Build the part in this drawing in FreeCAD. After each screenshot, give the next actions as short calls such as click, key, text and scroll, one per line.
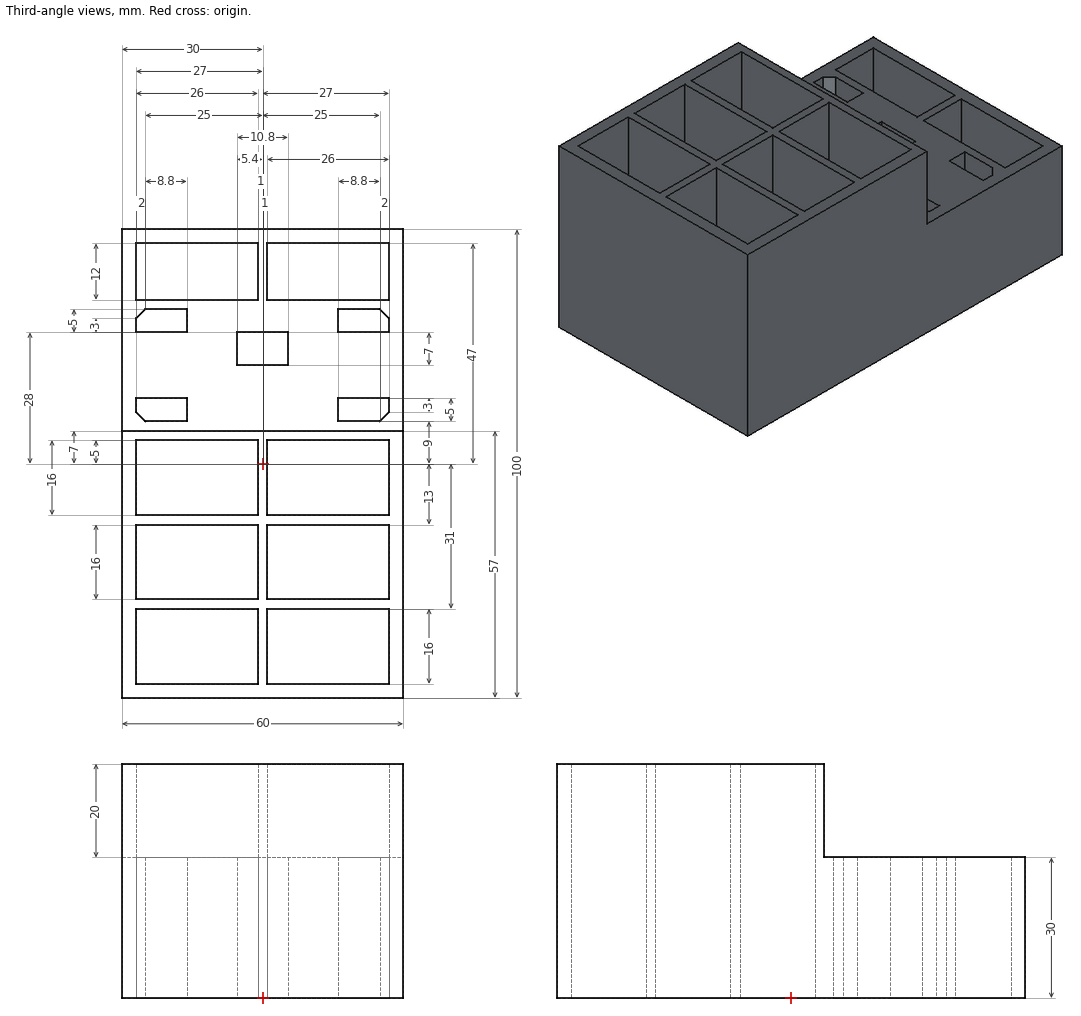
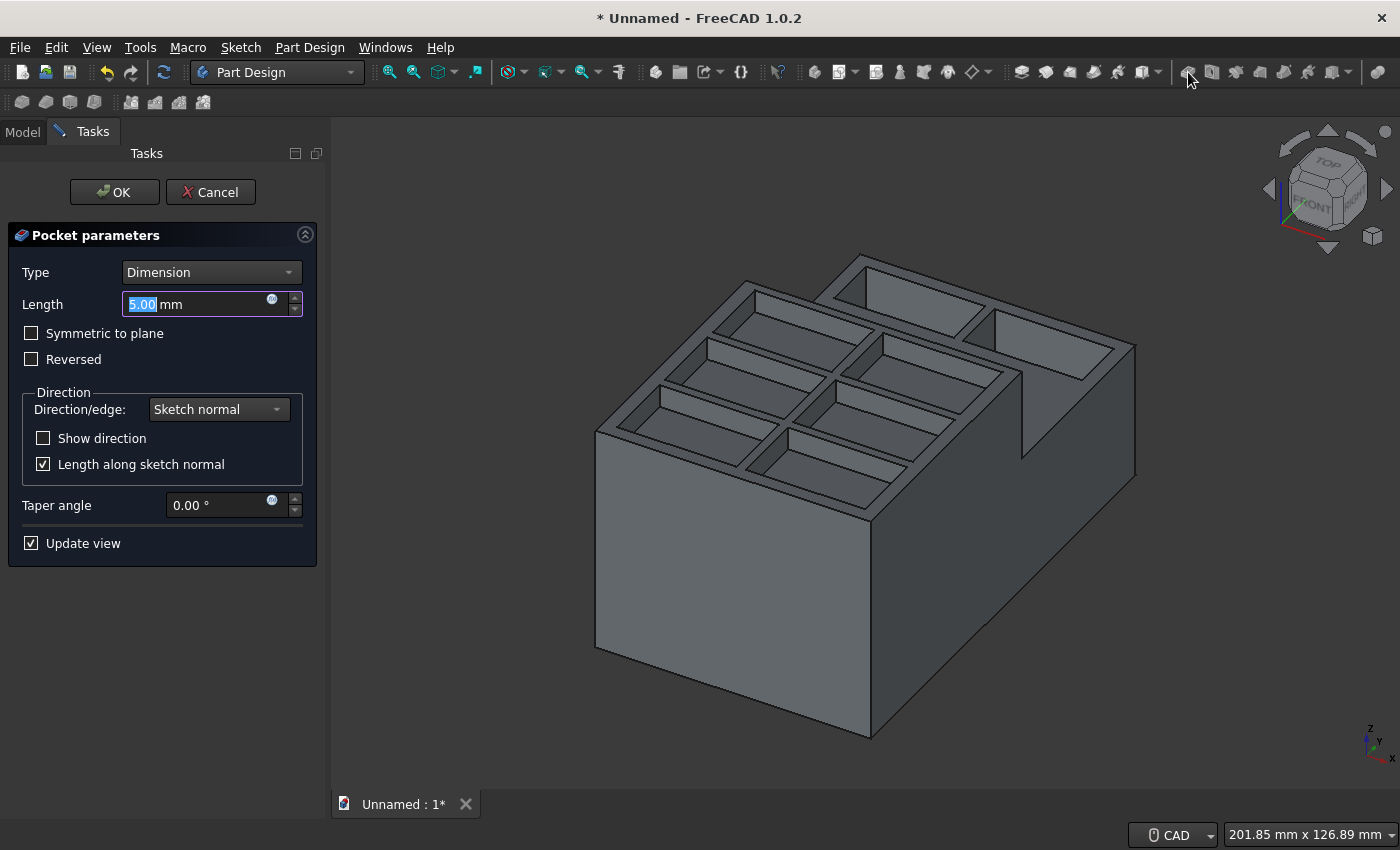
click(212, 272)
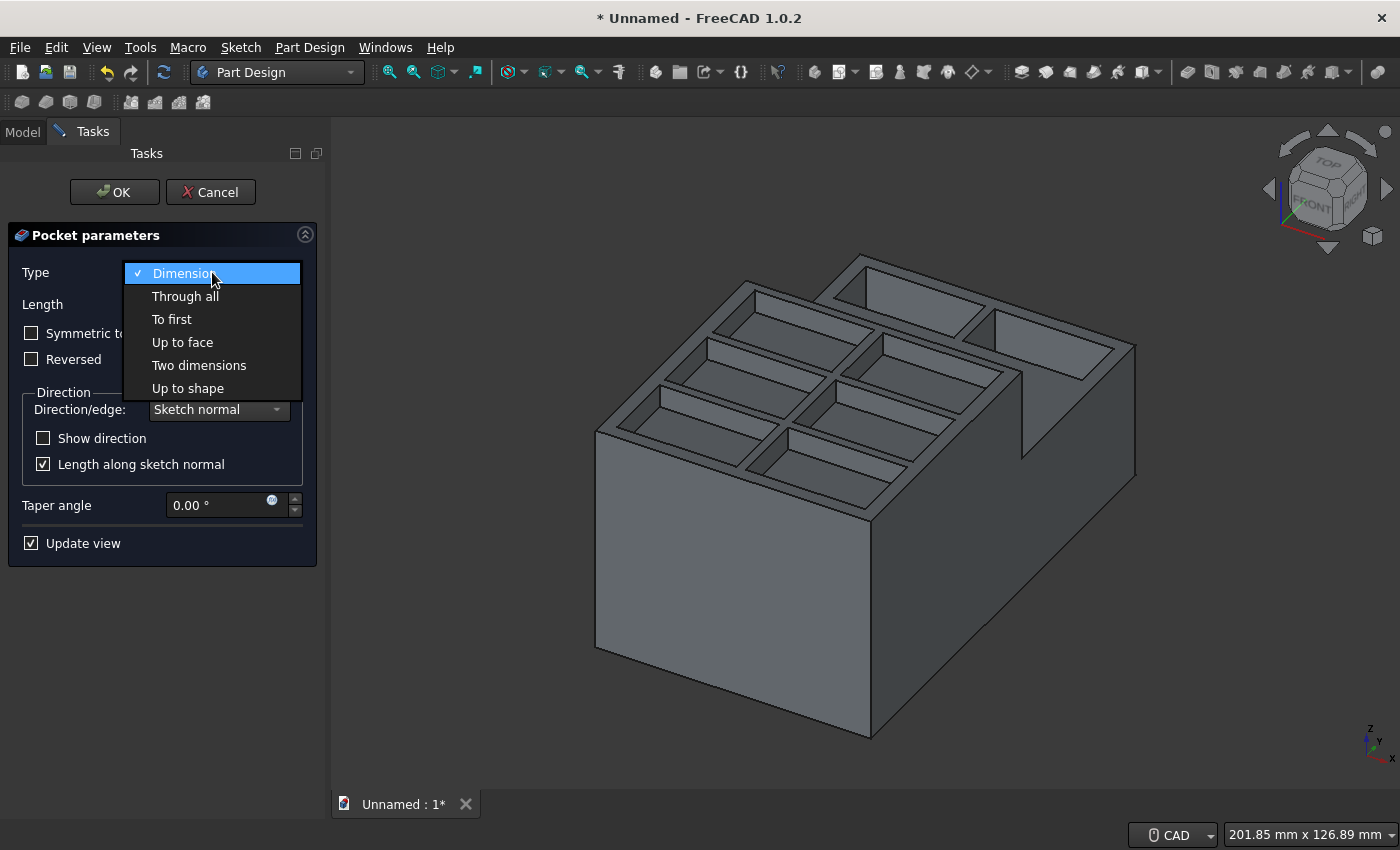
click(212, 296)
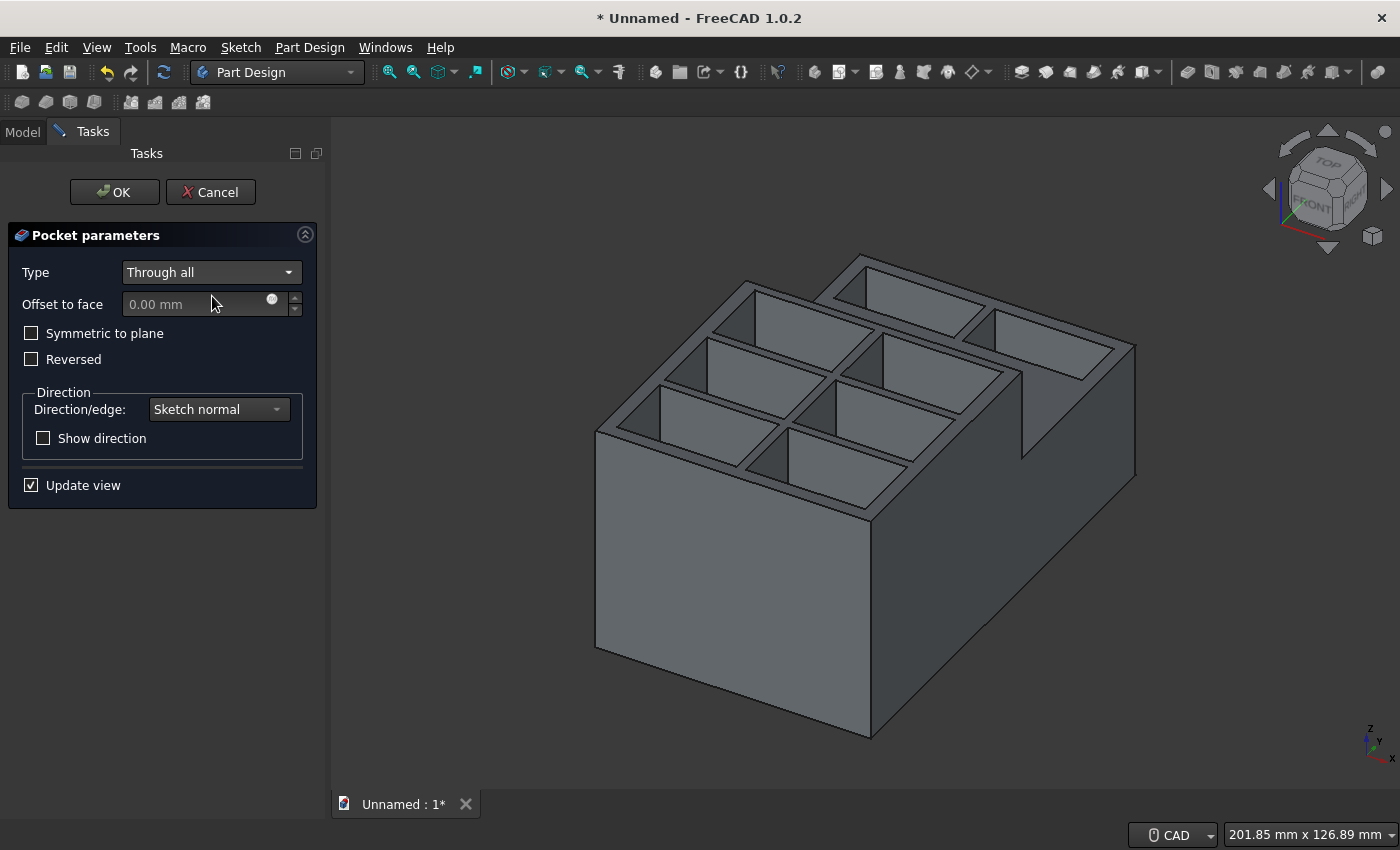
click(115, 192)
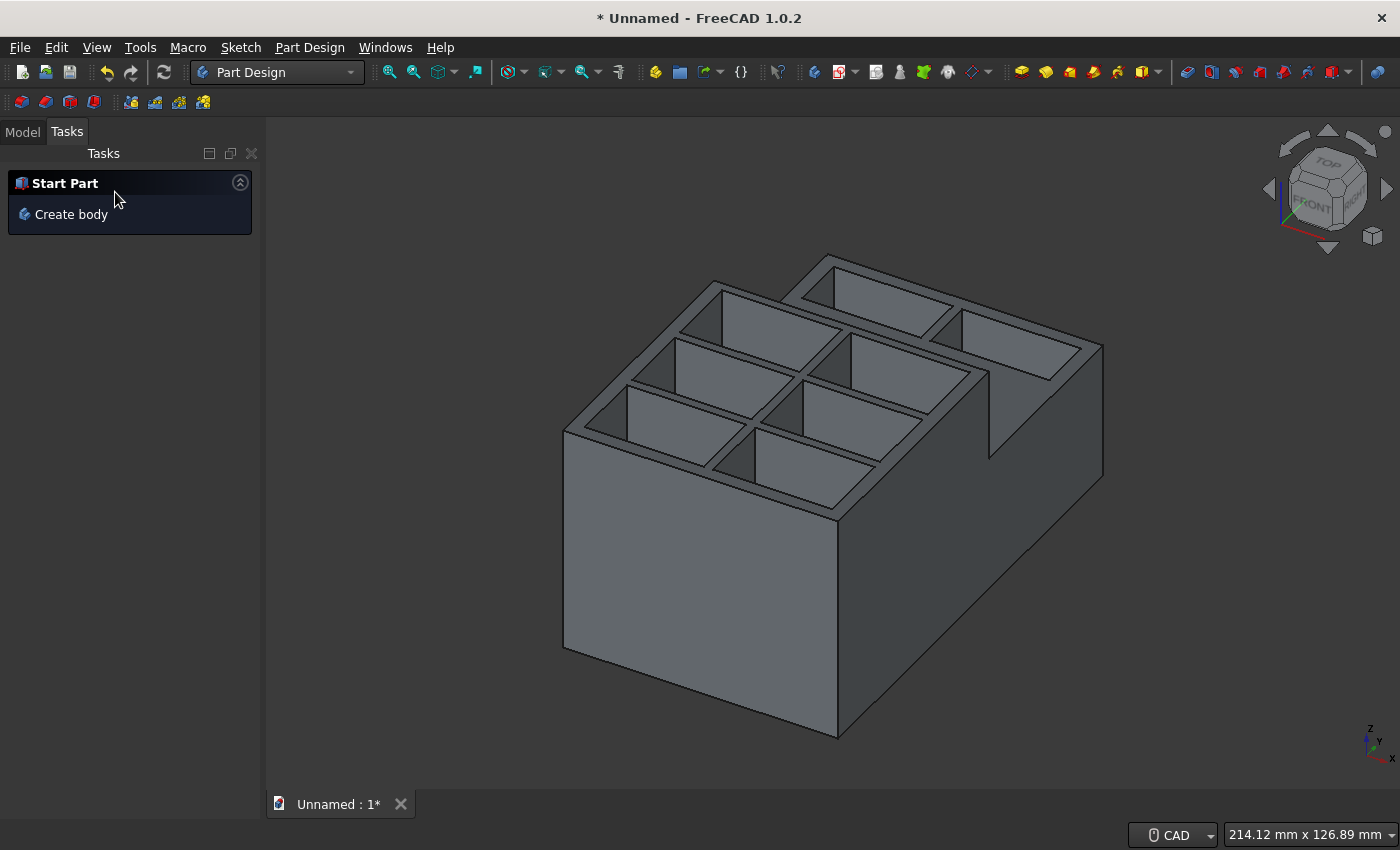
key(0)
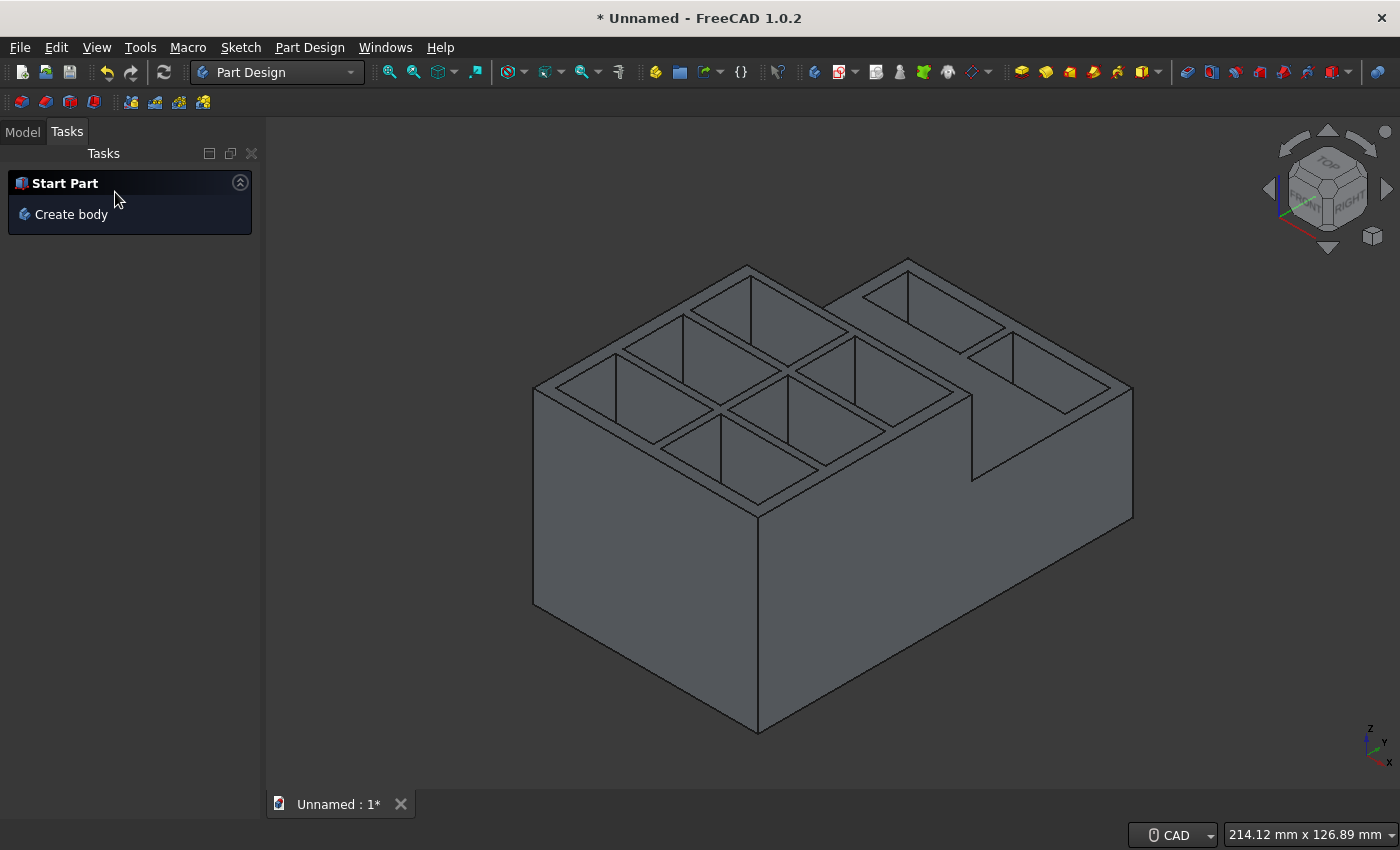
click(981, 419)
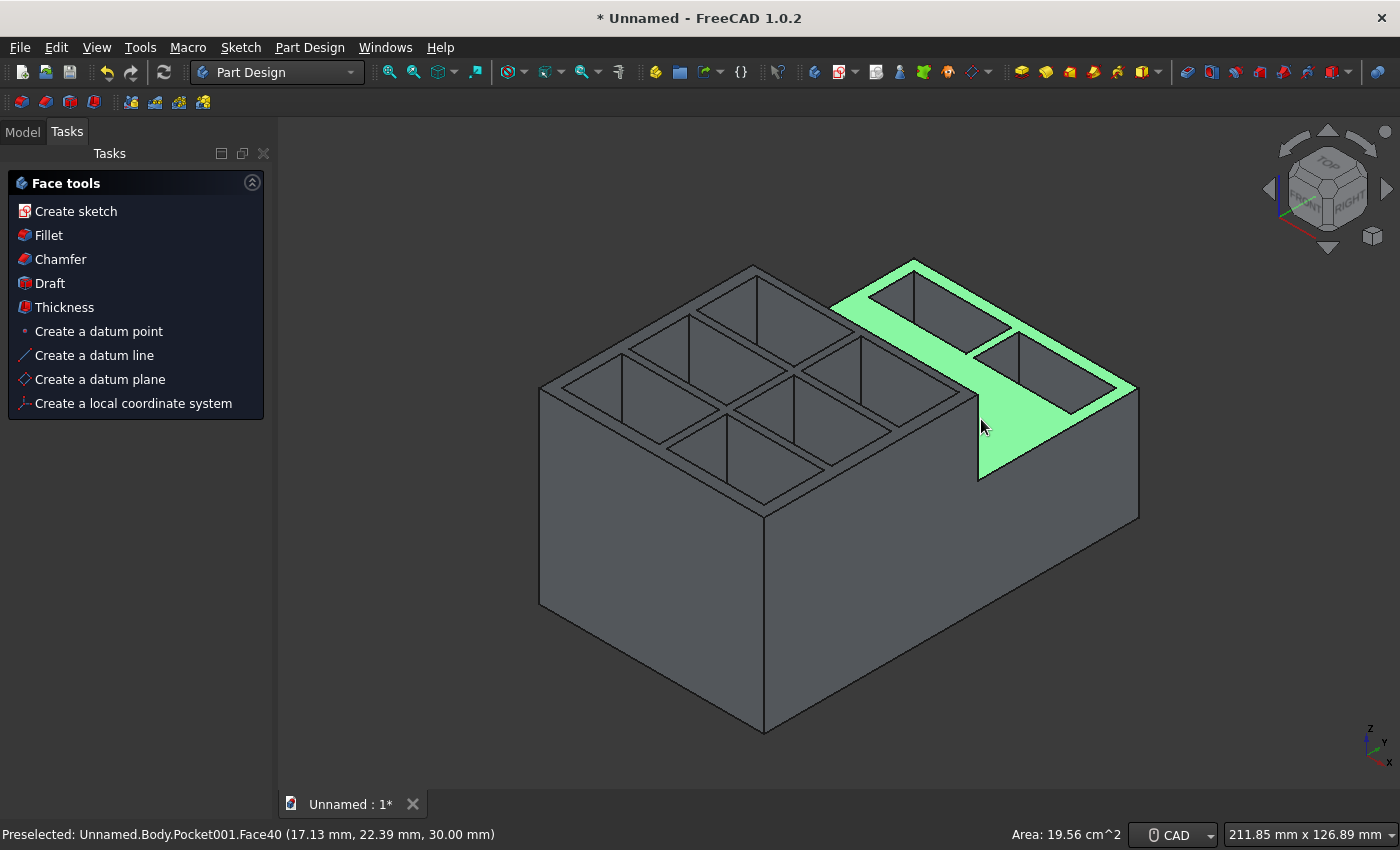
click(840, 72)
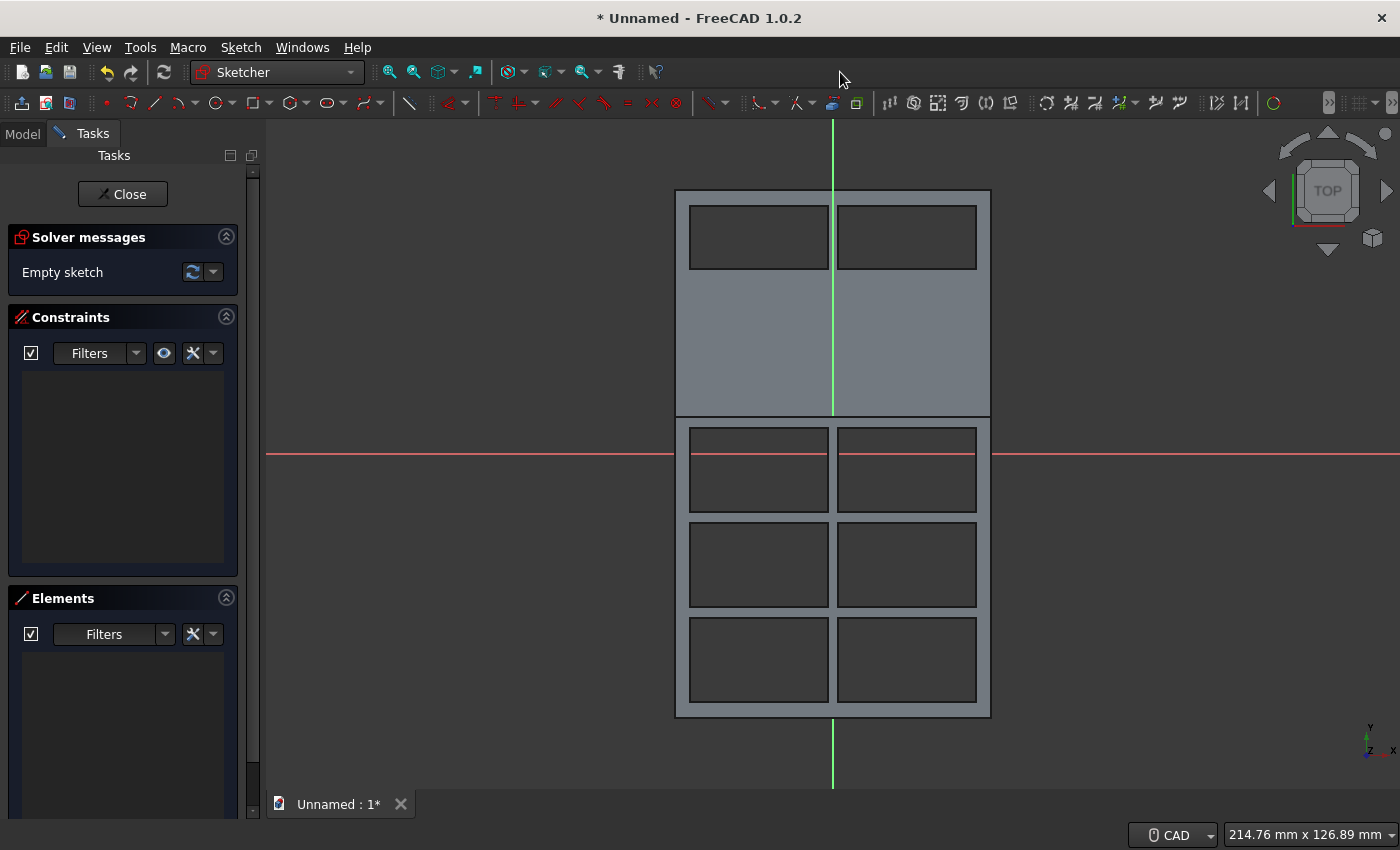
key(q)
key(s)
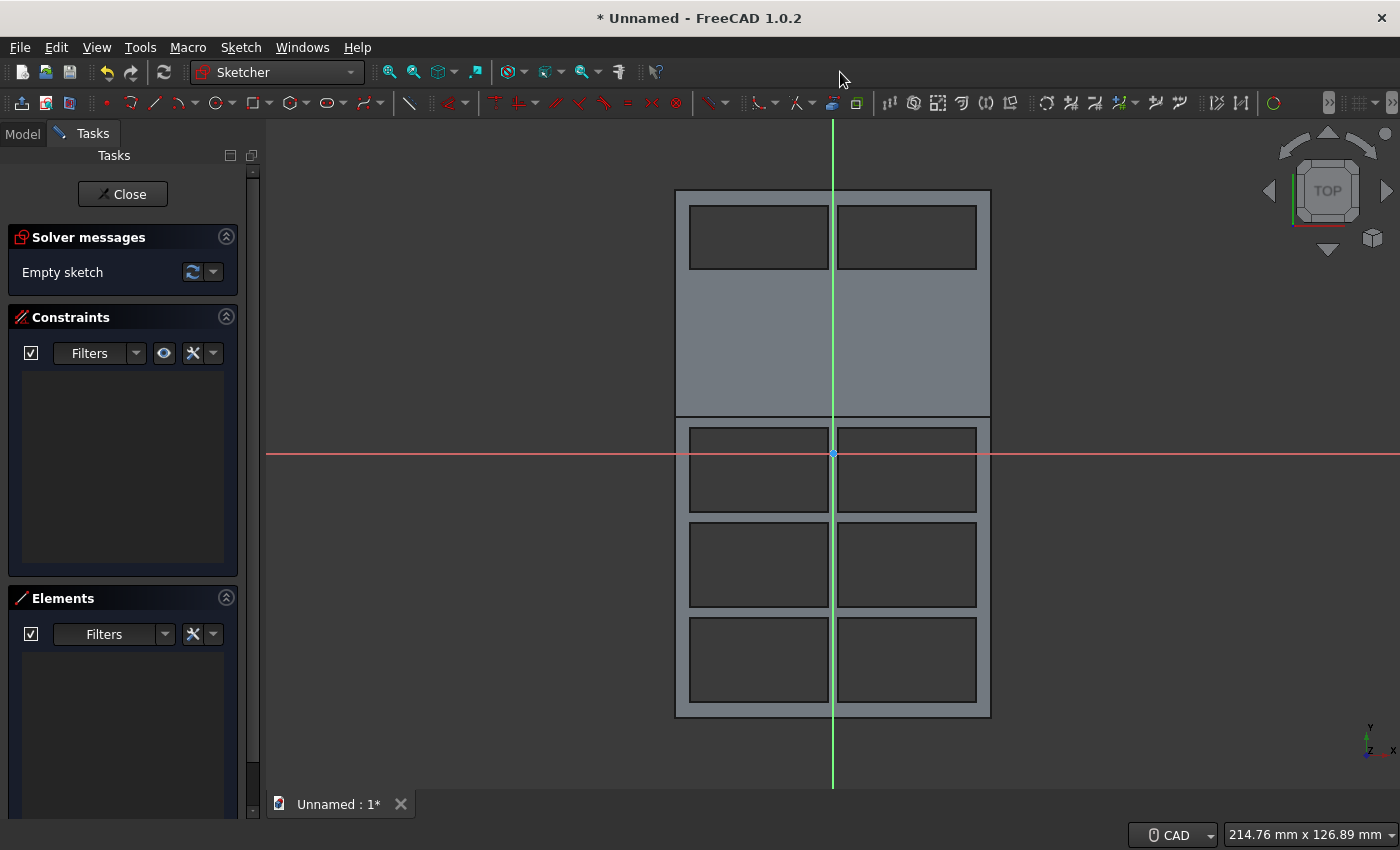
scroll(889, 296, up, 4)